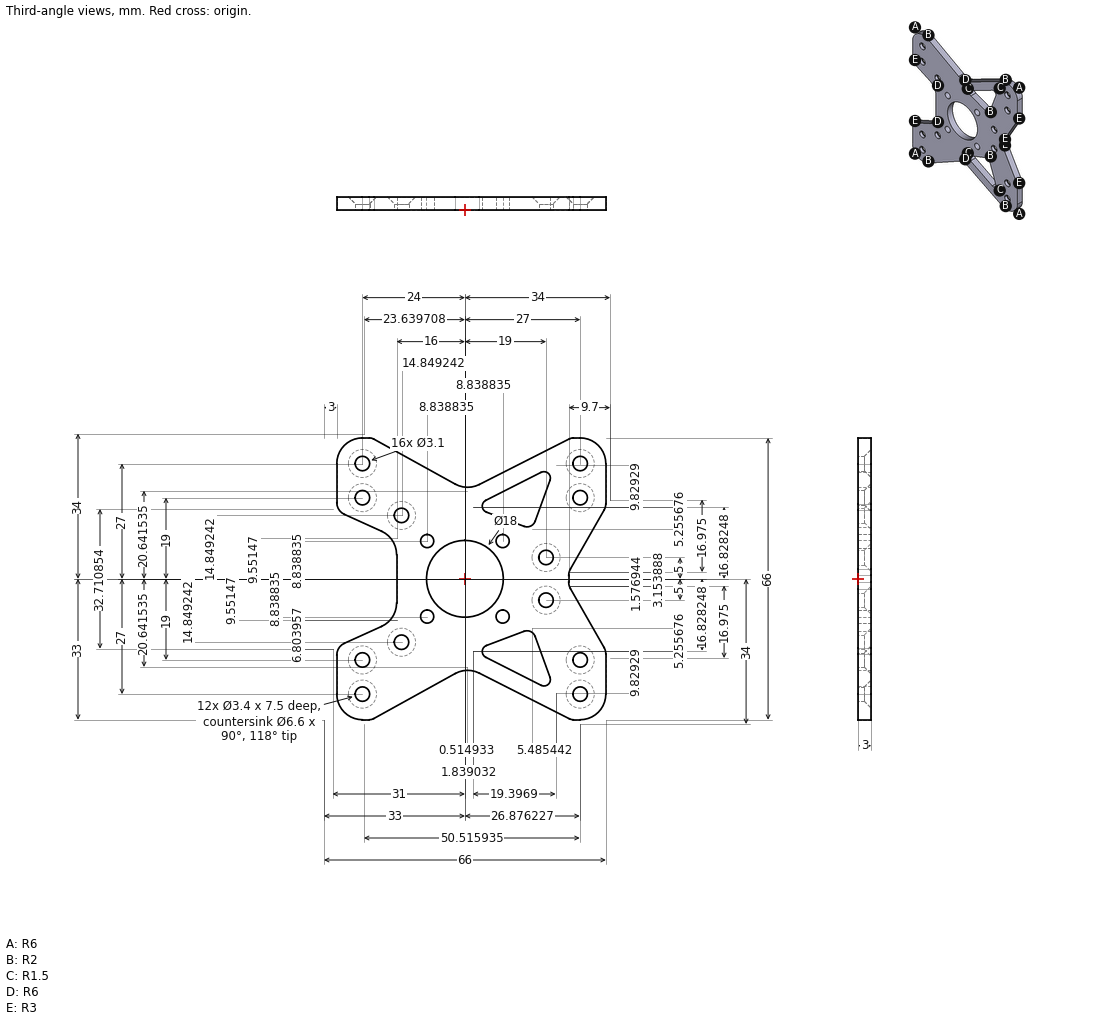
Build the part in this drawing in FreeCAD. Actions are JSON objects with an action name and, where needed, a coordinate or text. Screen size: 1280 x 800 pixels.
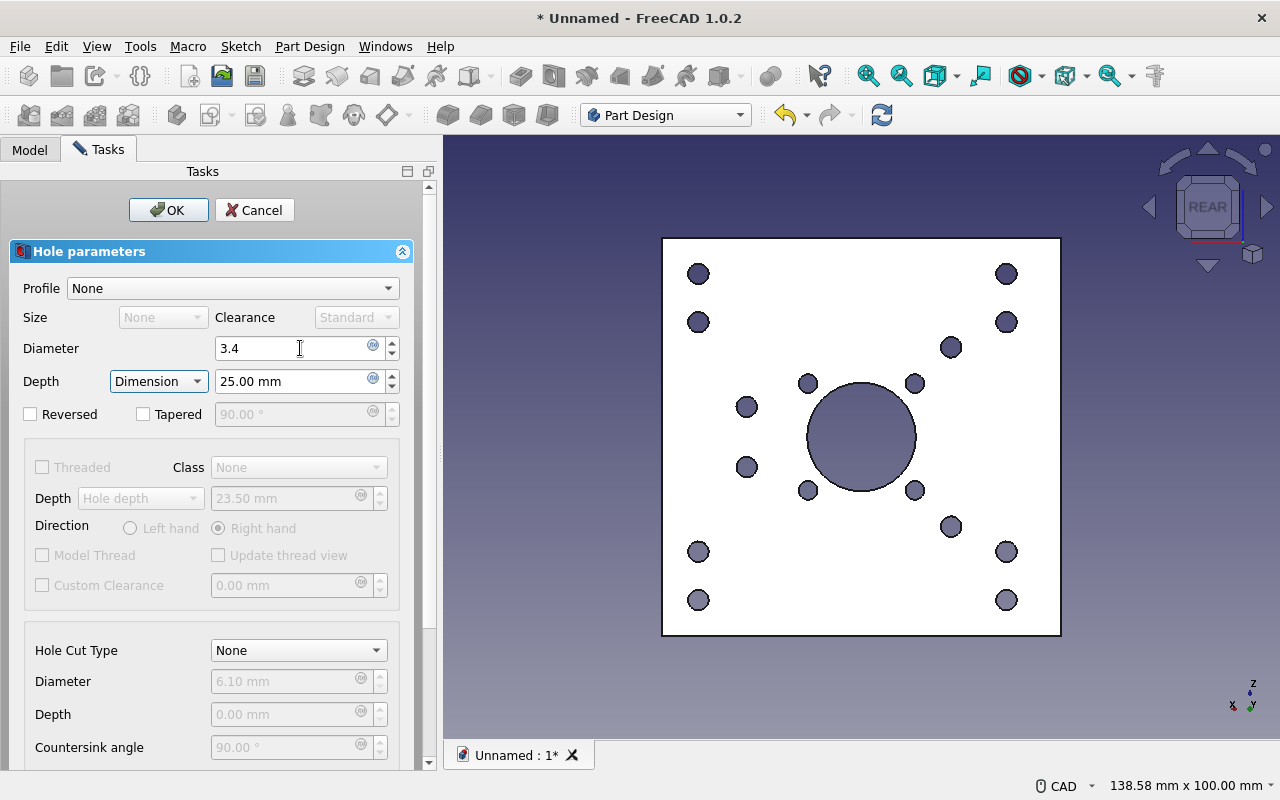
{"action": "triple_click", "coordinate": [300, 382]}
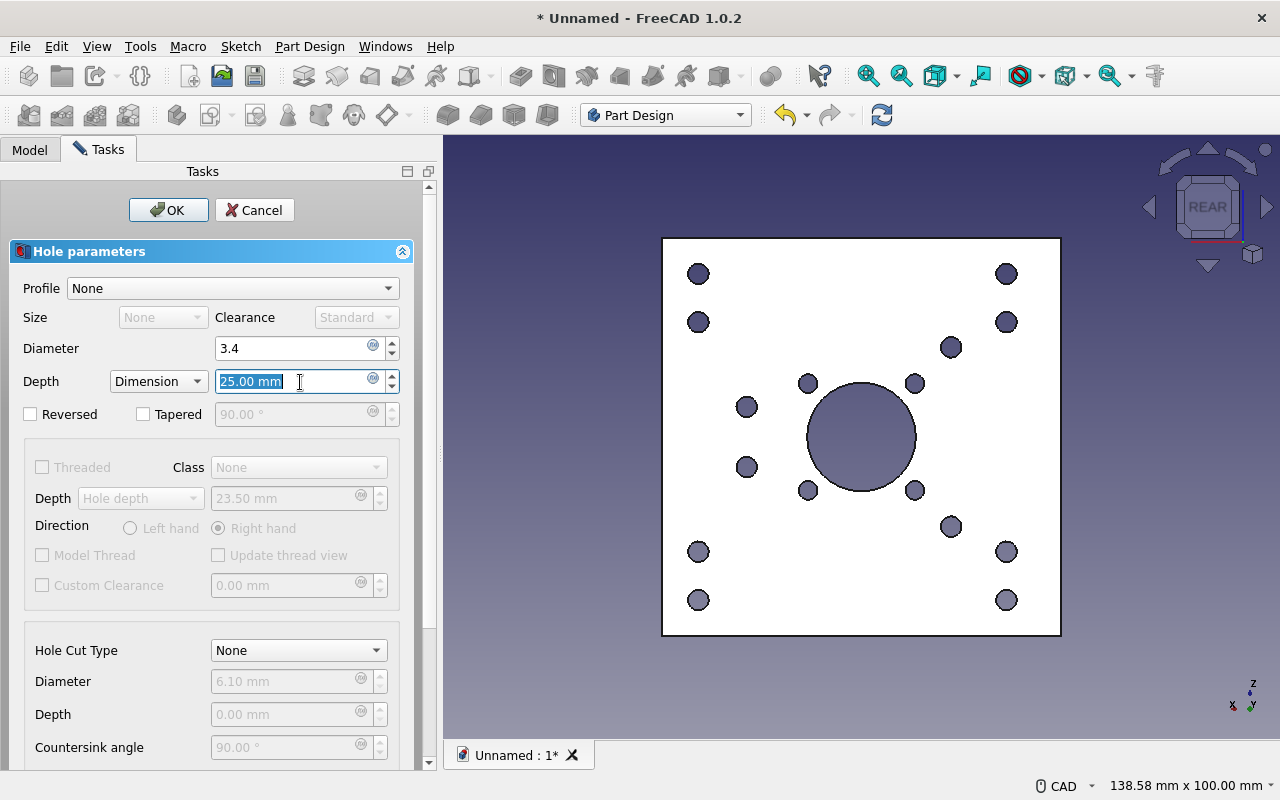
{"action": "type", "text": "7.5"}
{"action": "key", "text": "Tab"}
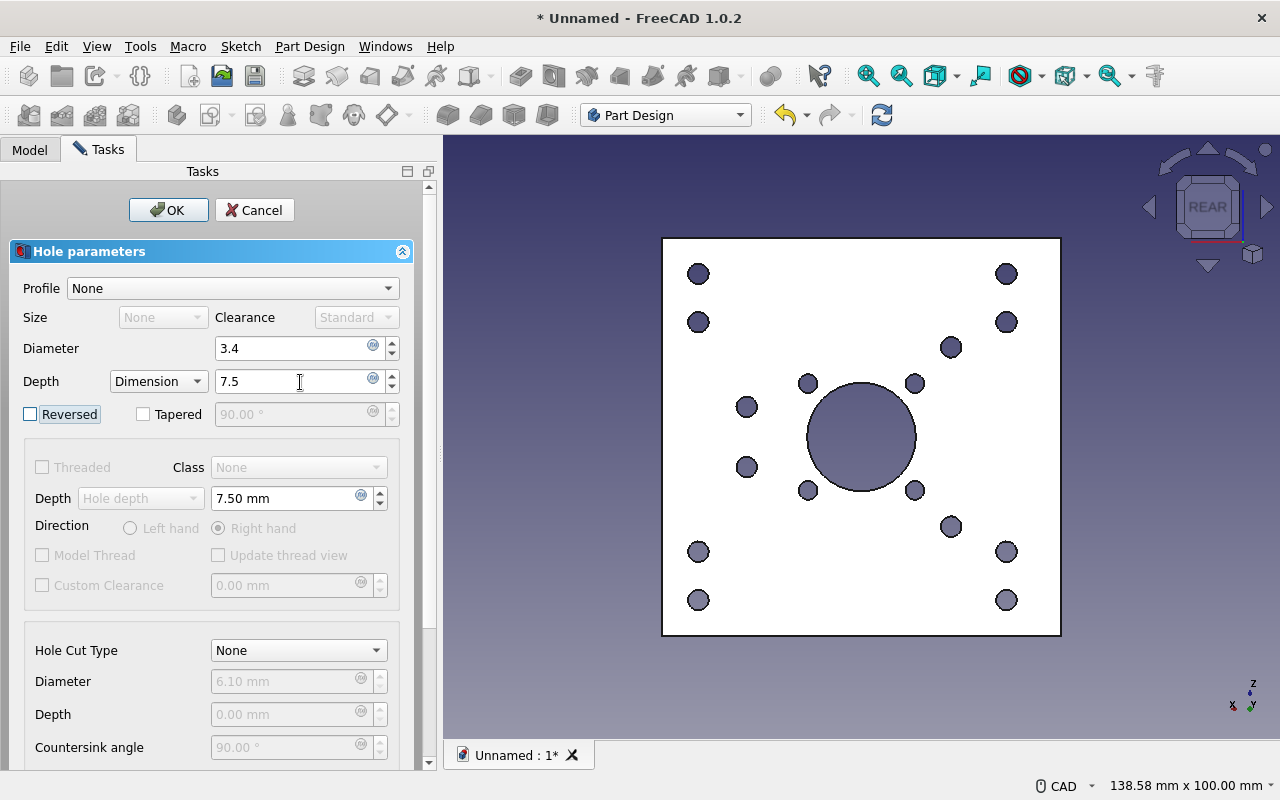
{"action": "left_click", "coordinate": [300, 650]}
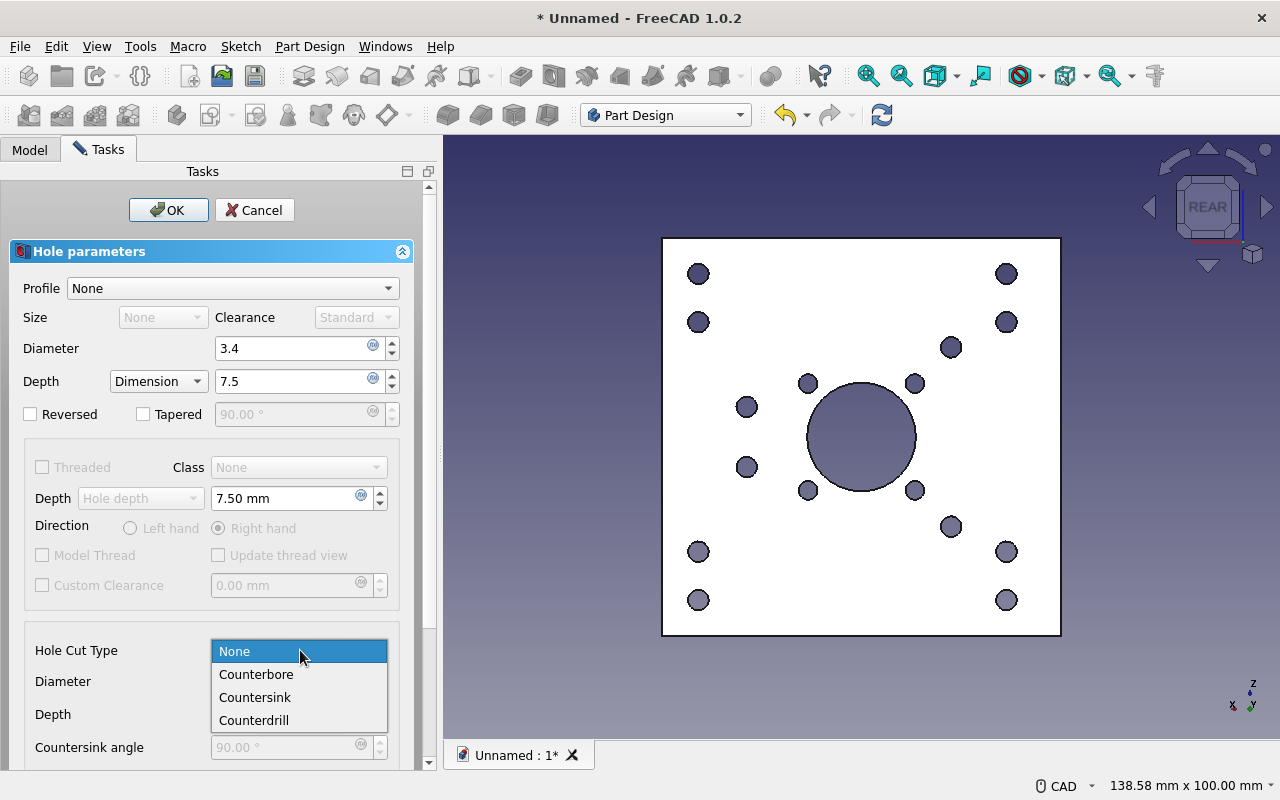
{"action": "left_click", "coordinate": [298, 698]}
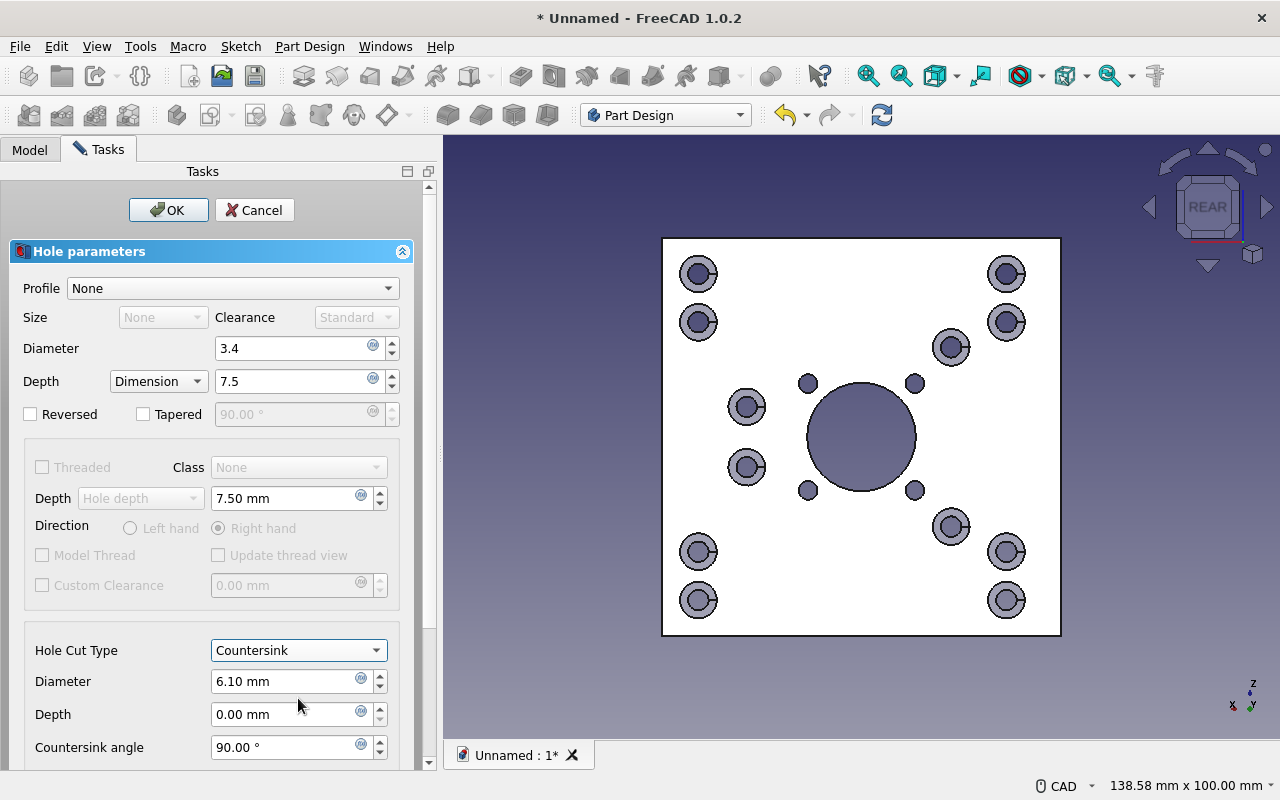
{"action": "triple_click", "coordinate": [292, 682]}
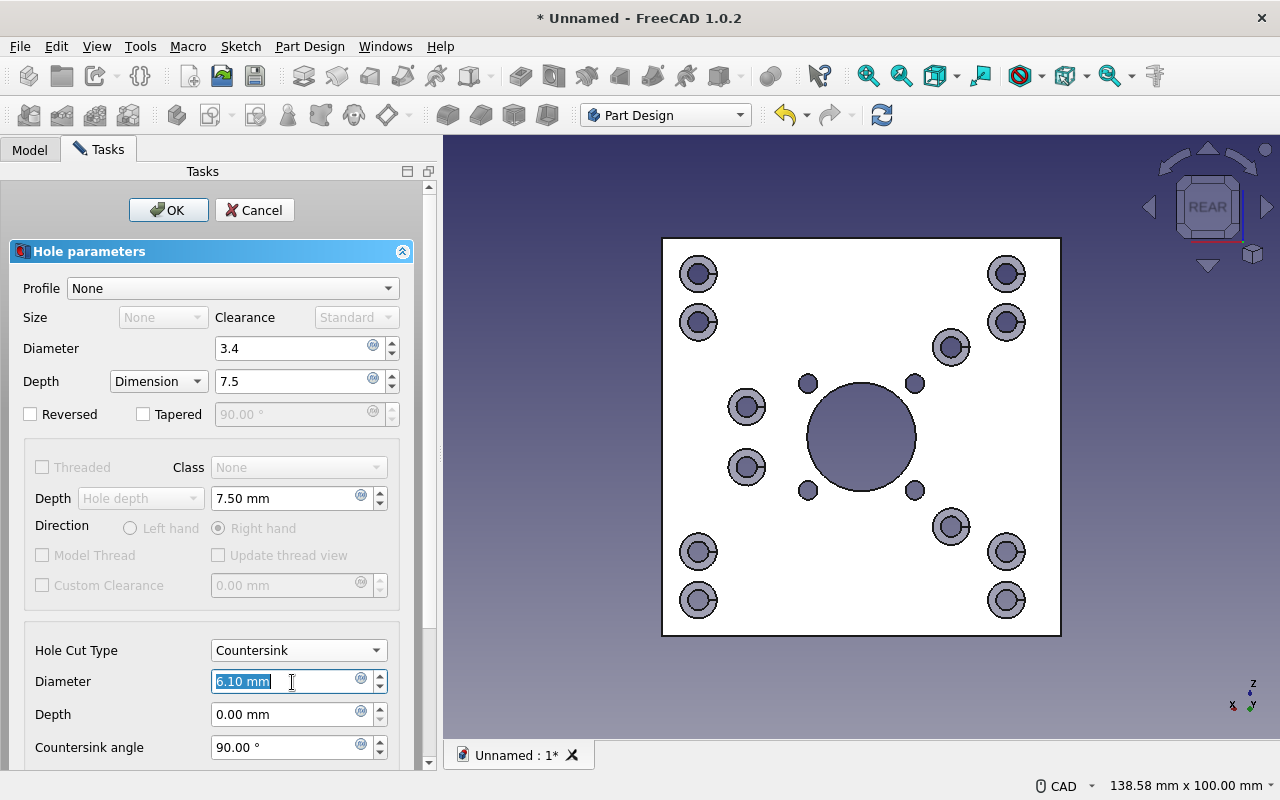
{"action": "type", "text": "6.6"}
{"action": "key", "text": "Tab"}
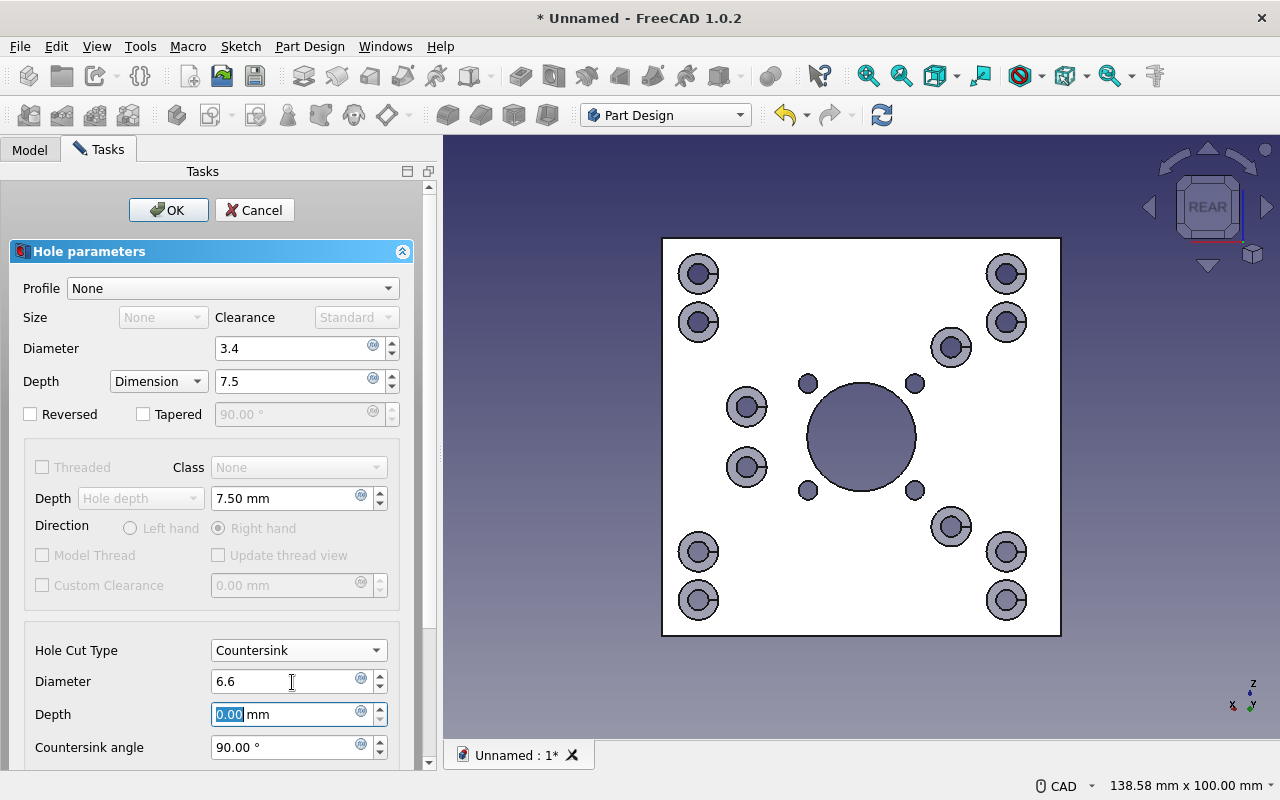
{"action": "left_click", "coordinate": [169, 210]}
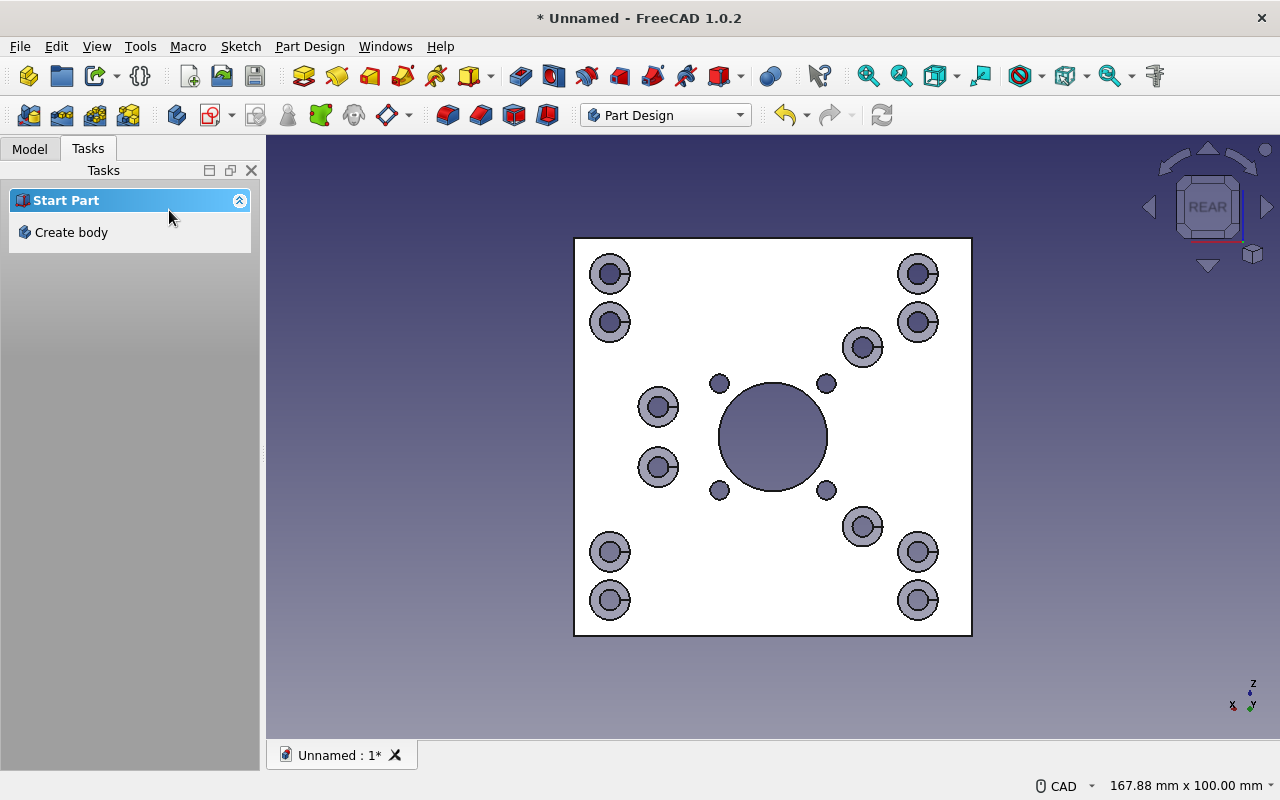
{"action": "left_click", "coordinate": [887, 436]}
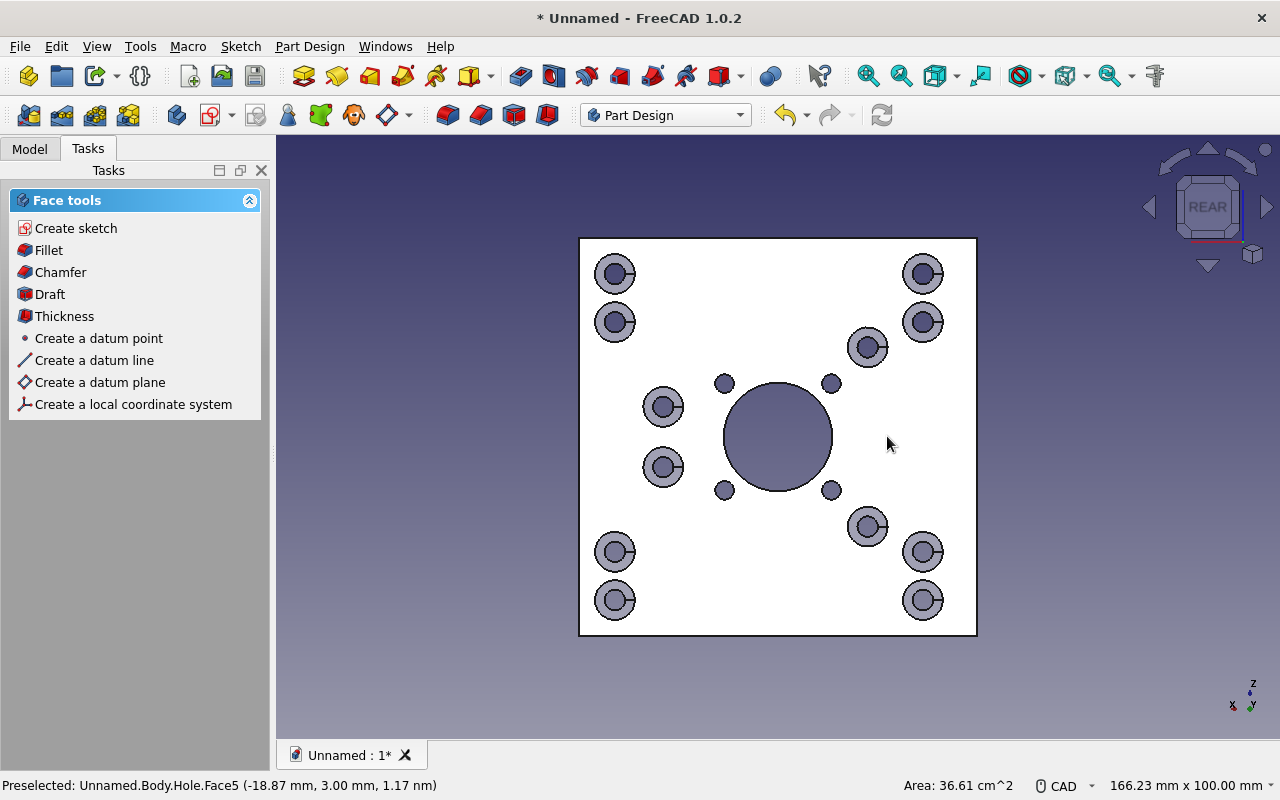
{"action": "left_click", "coordinate": [210, 116]}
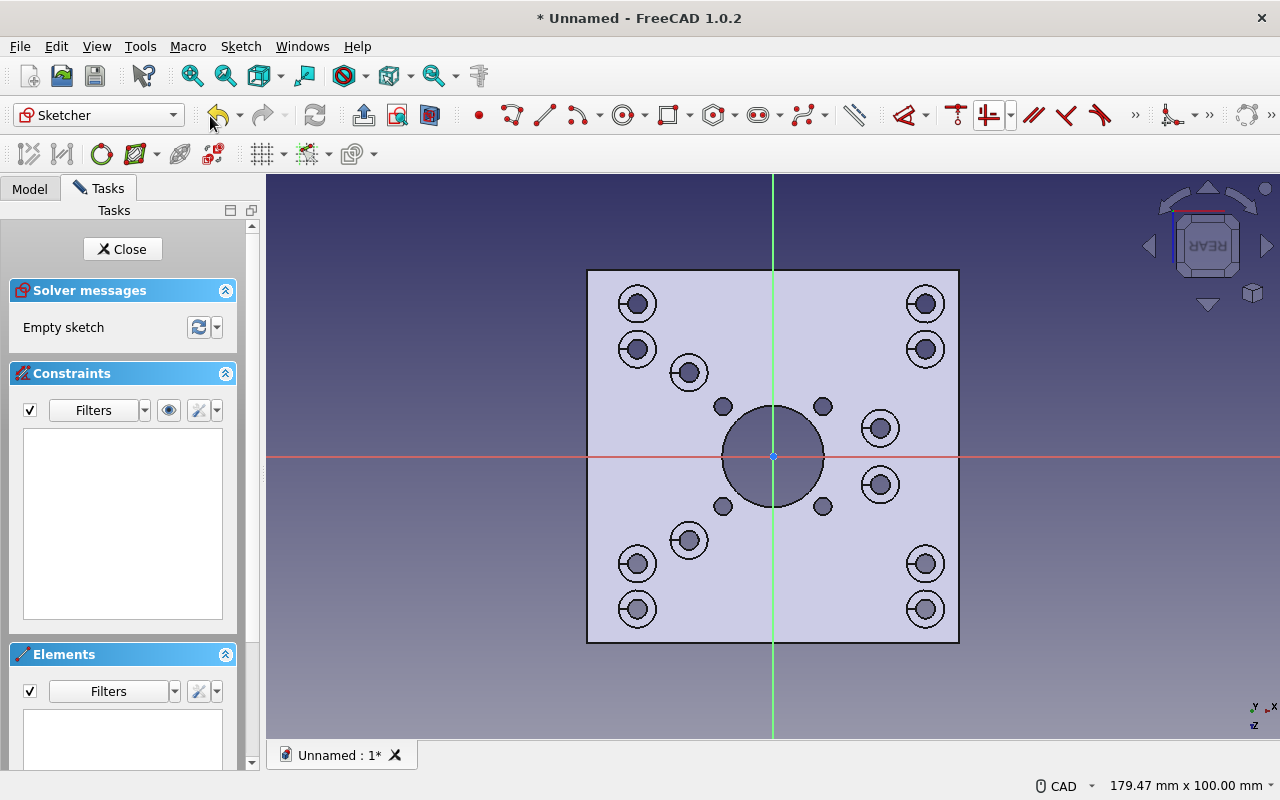
{"action": "left_click", "coordinate": [668, 116]}